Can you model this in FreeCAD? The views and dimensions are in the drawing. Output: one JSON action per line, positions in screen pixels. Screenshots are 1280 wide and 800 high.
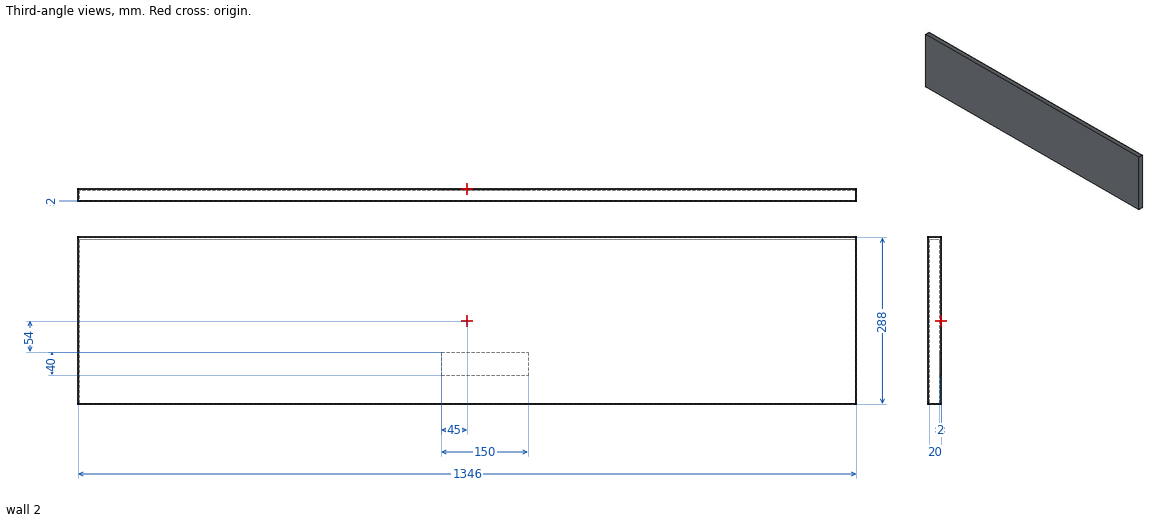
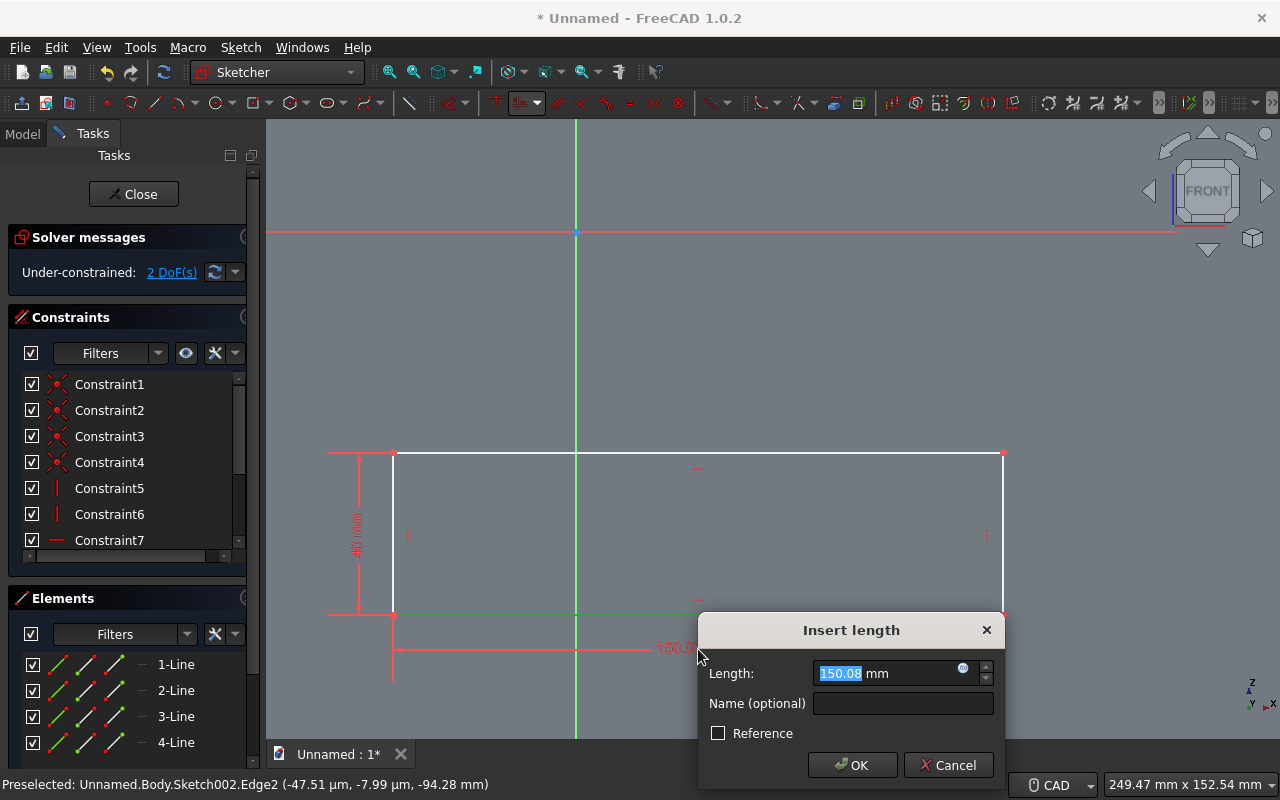
{"action": "type", "text": "150"}
{"action": "key", "text": "Return"}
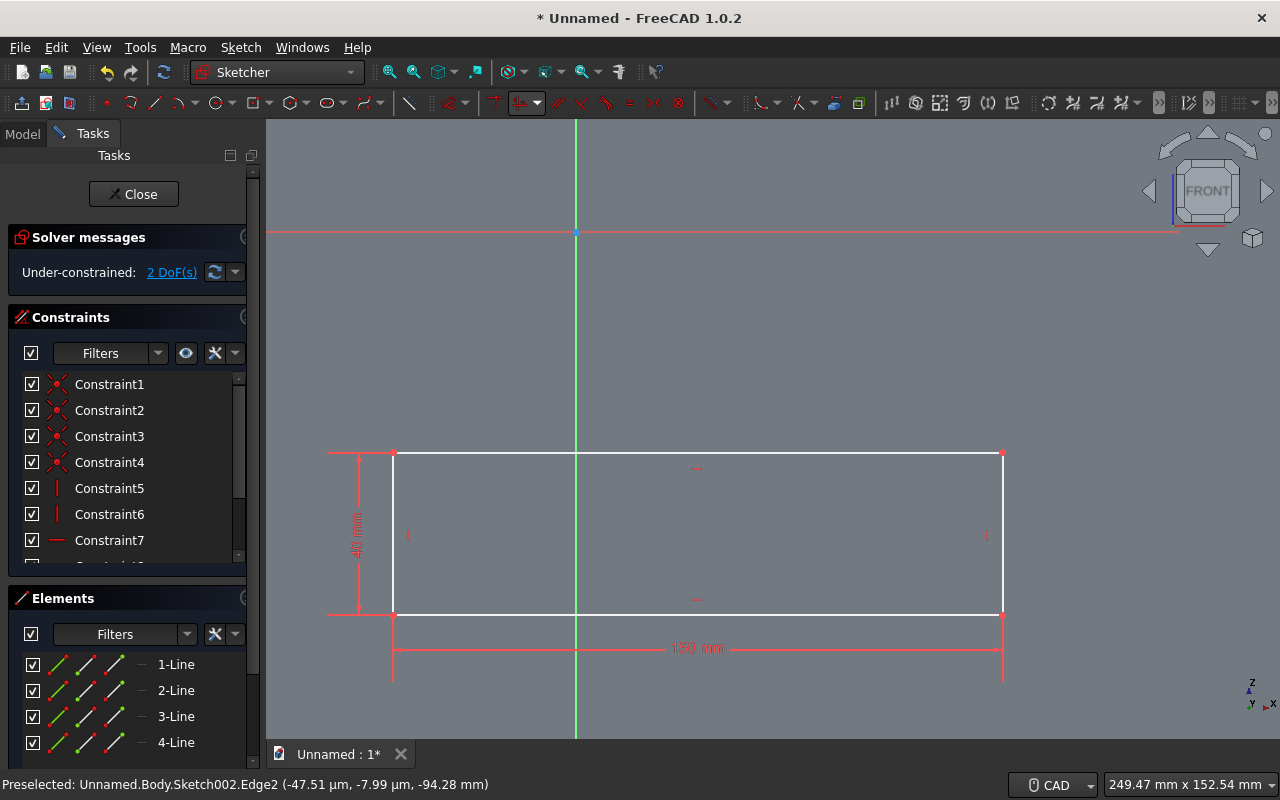
{"action": "left_click", "coordinate": [393, 453]}
{"action": "left_click", "coordinate": [485, 198]}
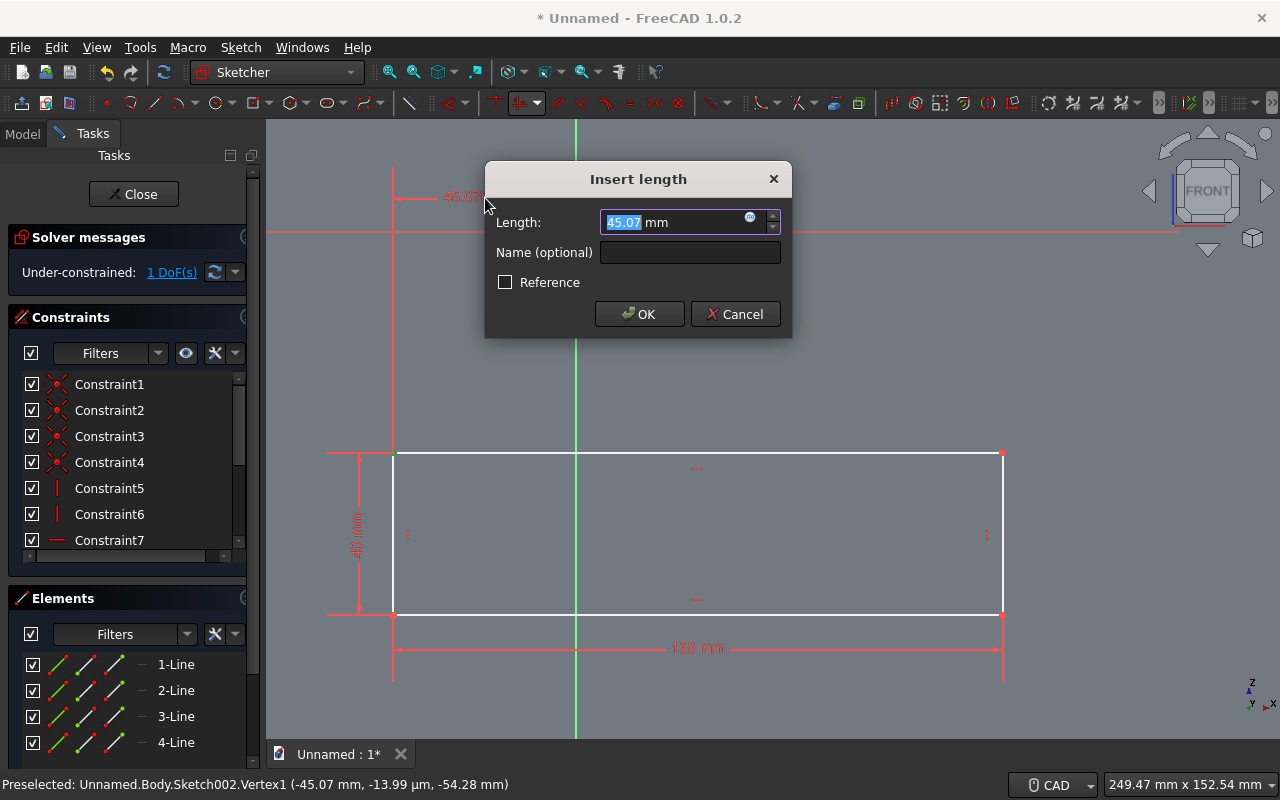
{"action": "type", "text": "45"}
{"action": "key", "text": "Return"}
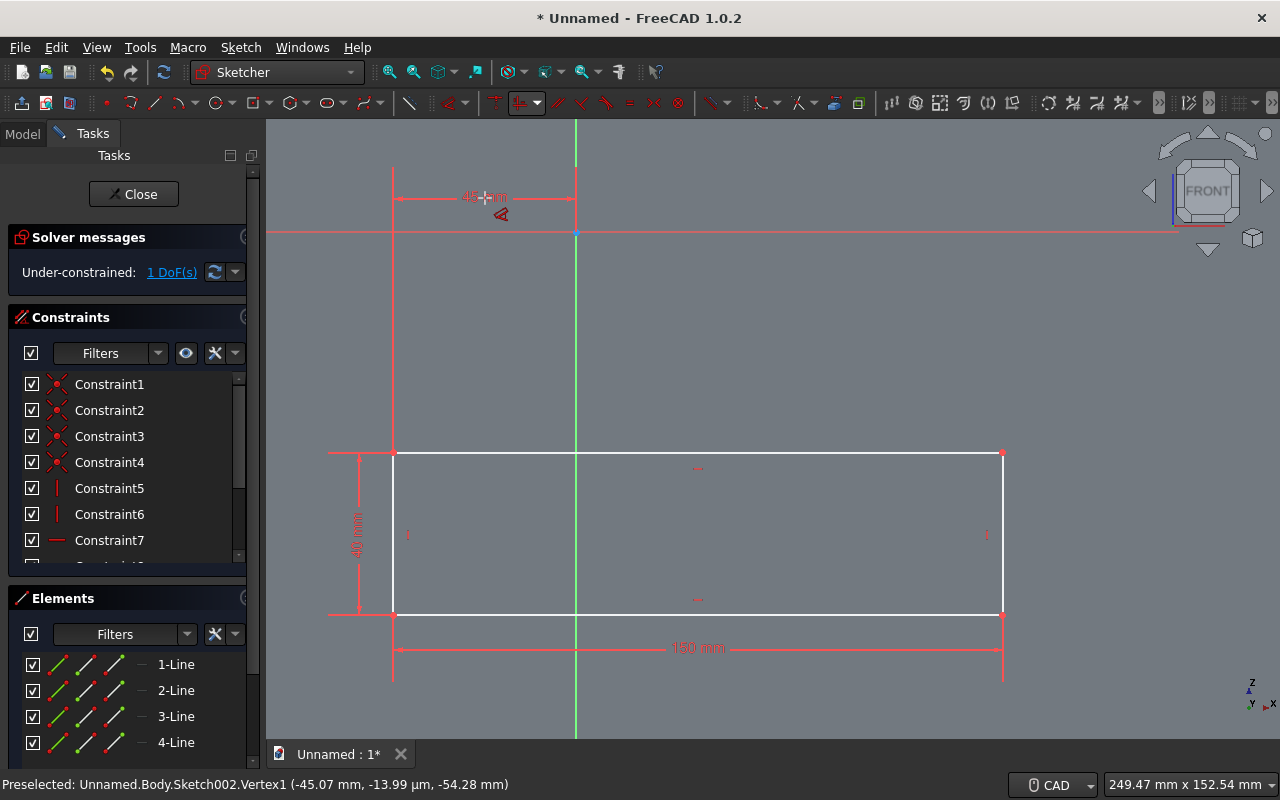
{"action": "left_click", "coordinate": [393, 453]}
{"action": "left_click", "coordinate": [359, 342]}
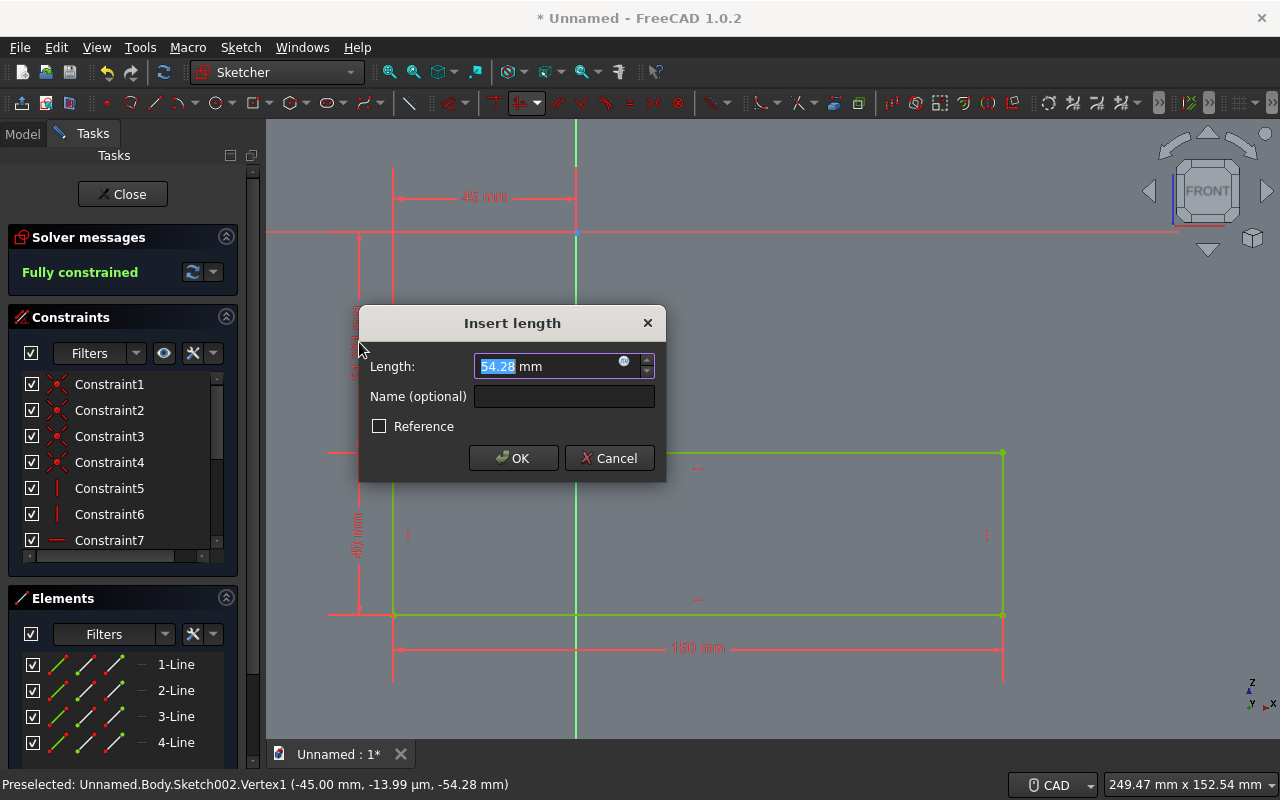
{"action": "type", "text": "54"}
{"action": "key", "text": "Return"}
{"action": "key", "text": "Escape"}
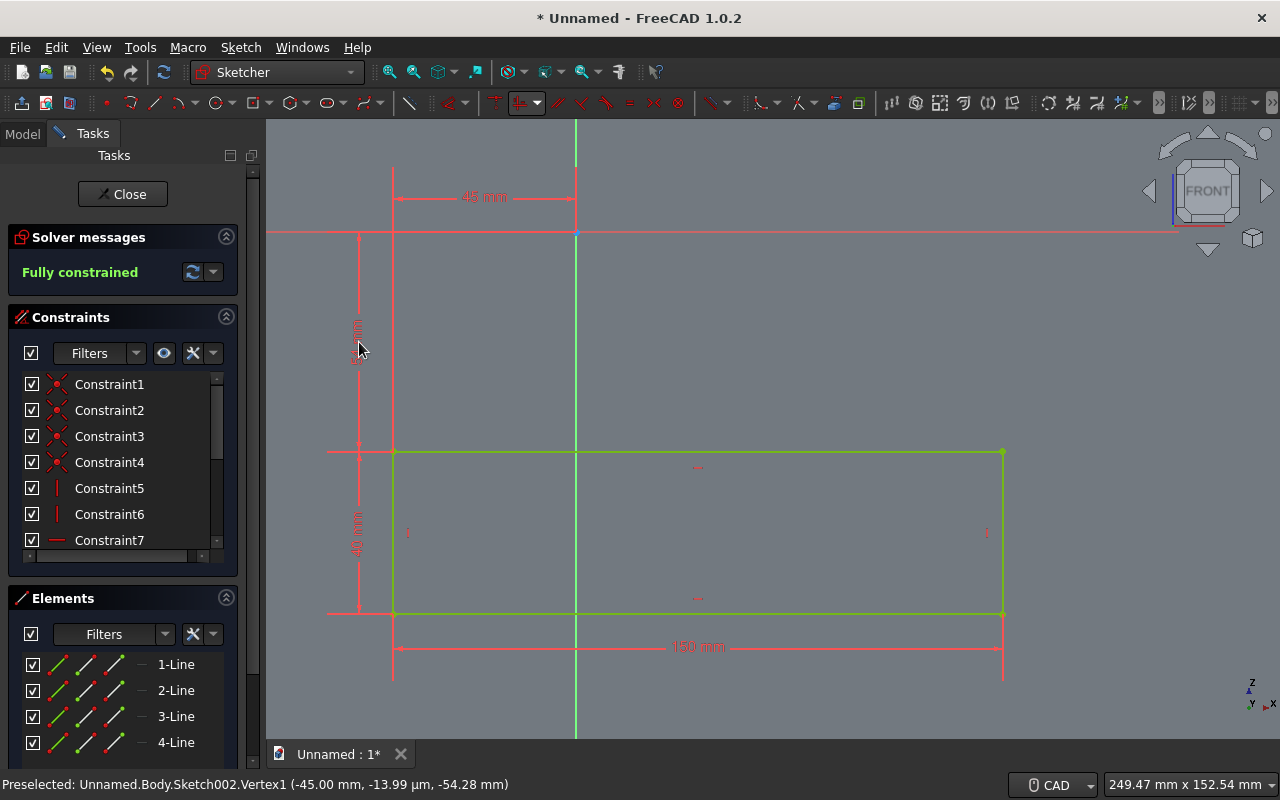
{"action": "left_click", "coordinate": [123, 194]}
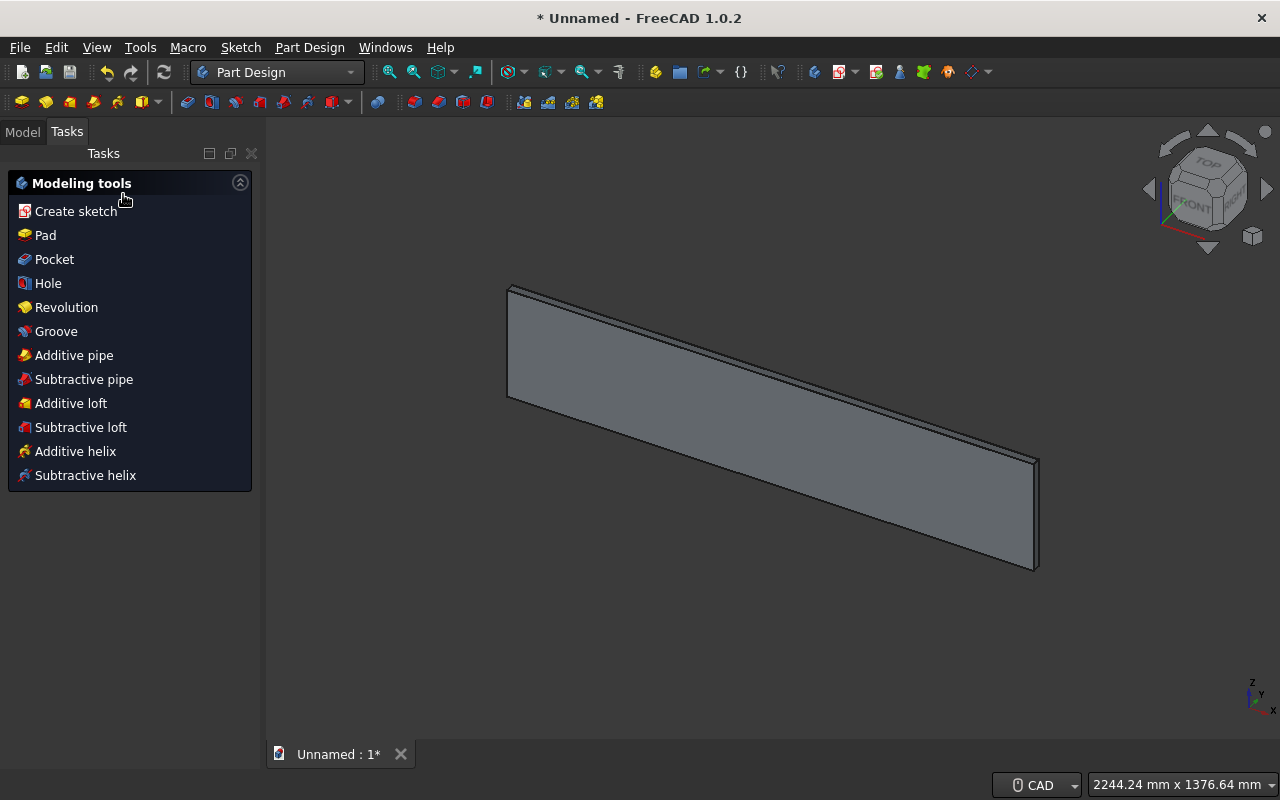
{"action": "left_click", "coordinate": [188, 102]}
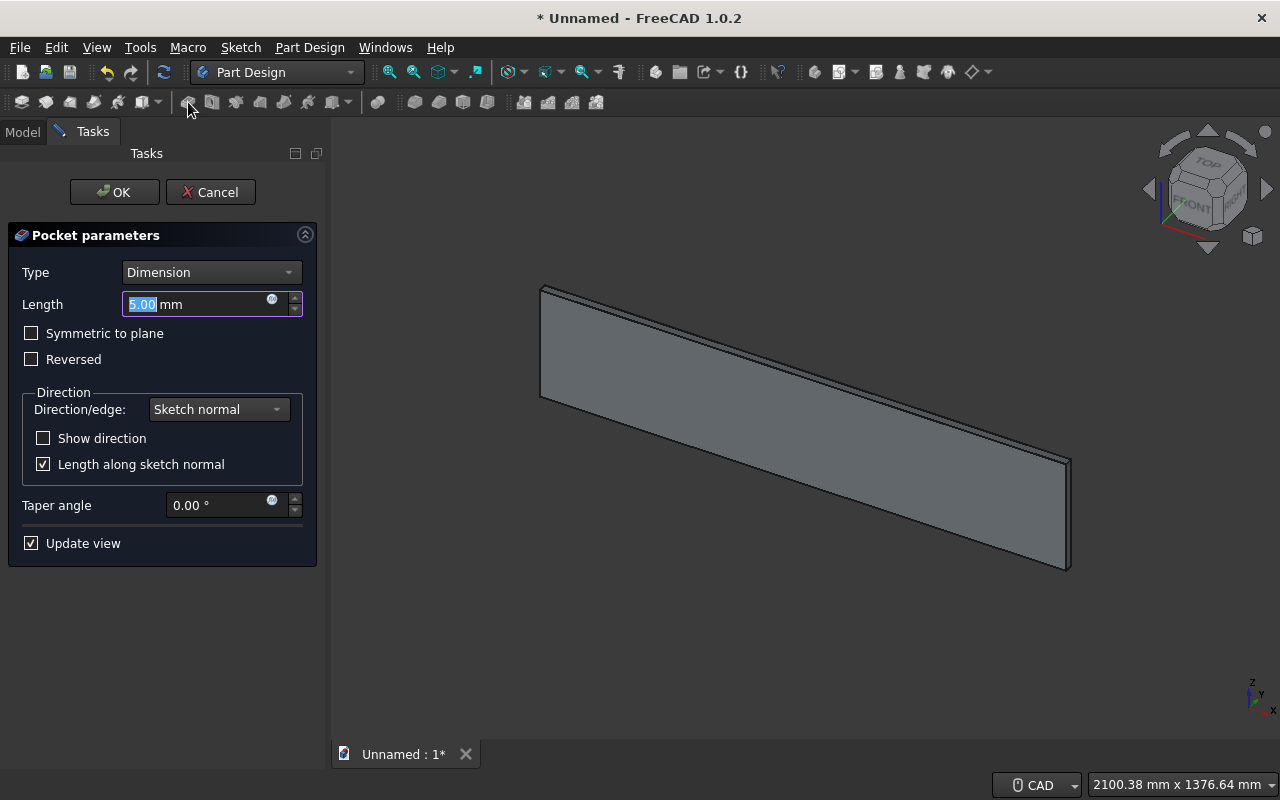
{"action": "type", "text": "2"}
{"action": "key", "text": "Tab"}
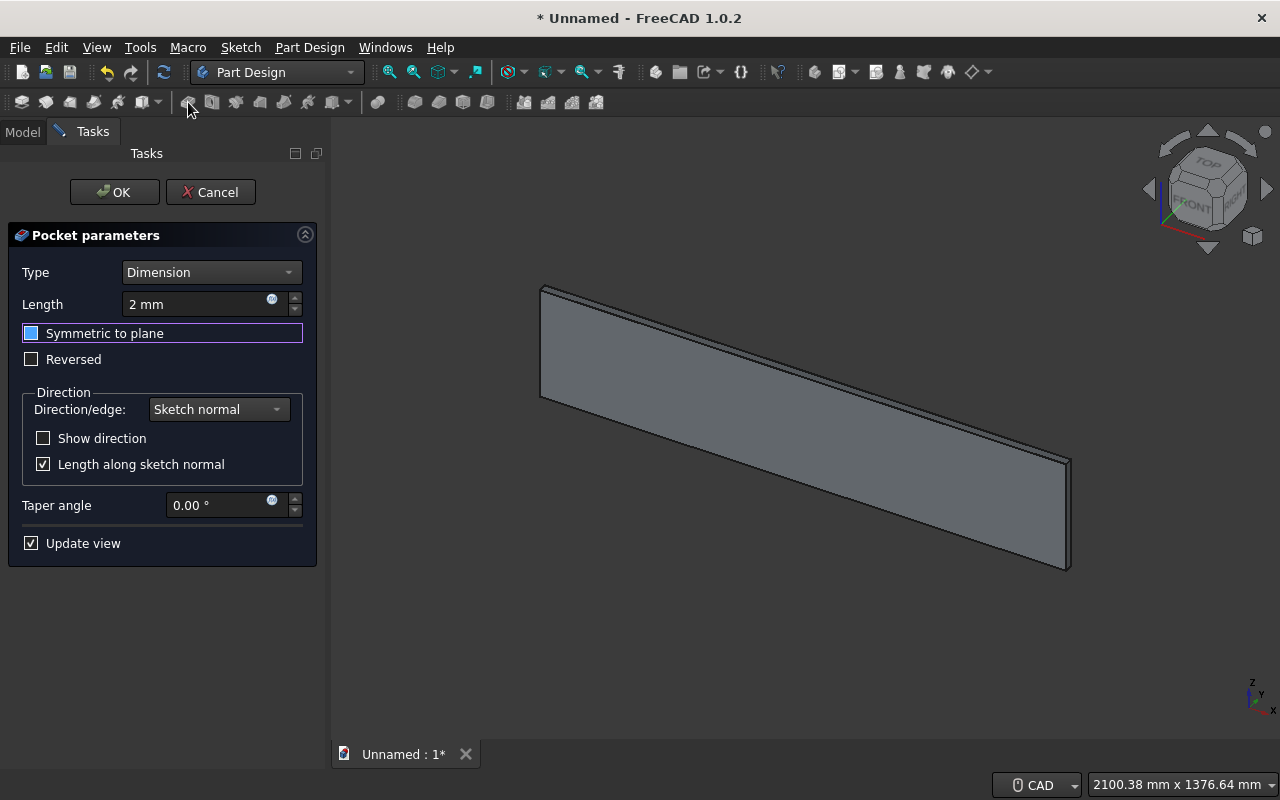
{"action": "left_click", "coordinate": [30, 359]}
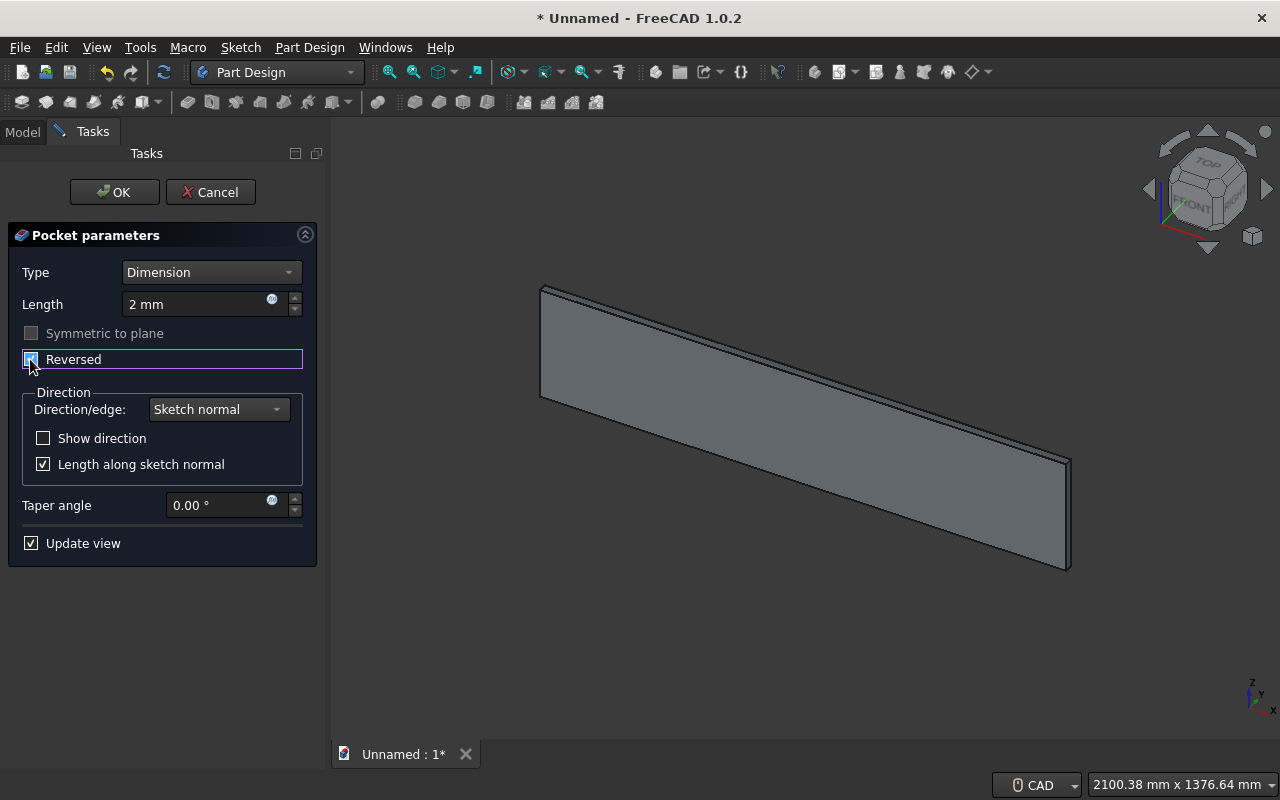
{"action": "left_click", "coordinate": [115, 192]}